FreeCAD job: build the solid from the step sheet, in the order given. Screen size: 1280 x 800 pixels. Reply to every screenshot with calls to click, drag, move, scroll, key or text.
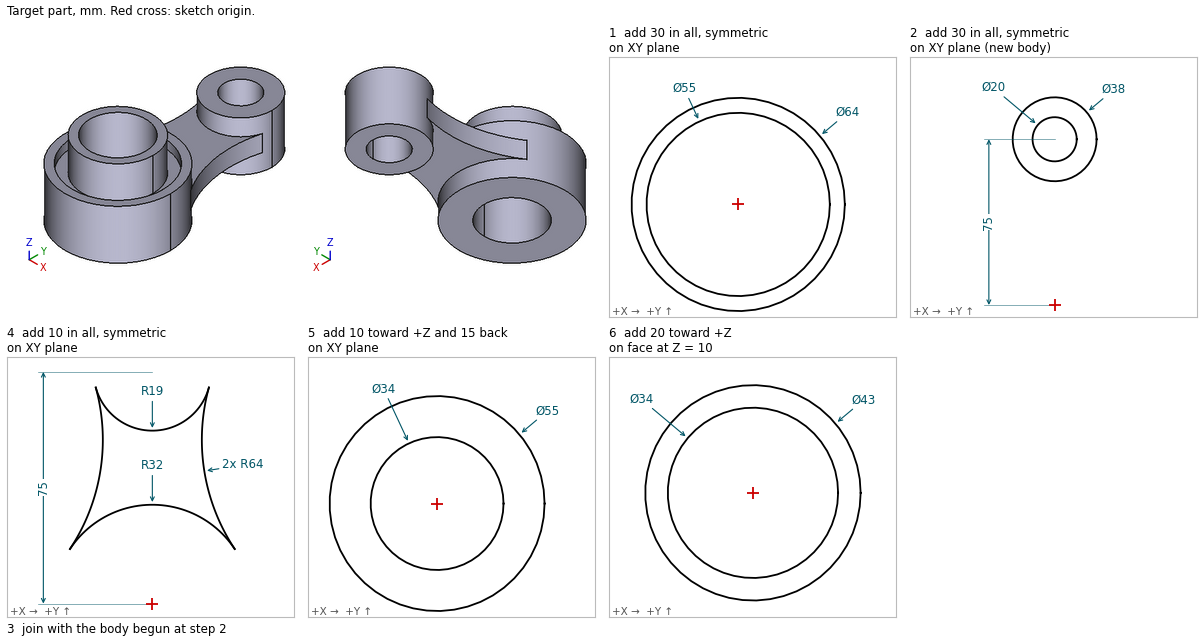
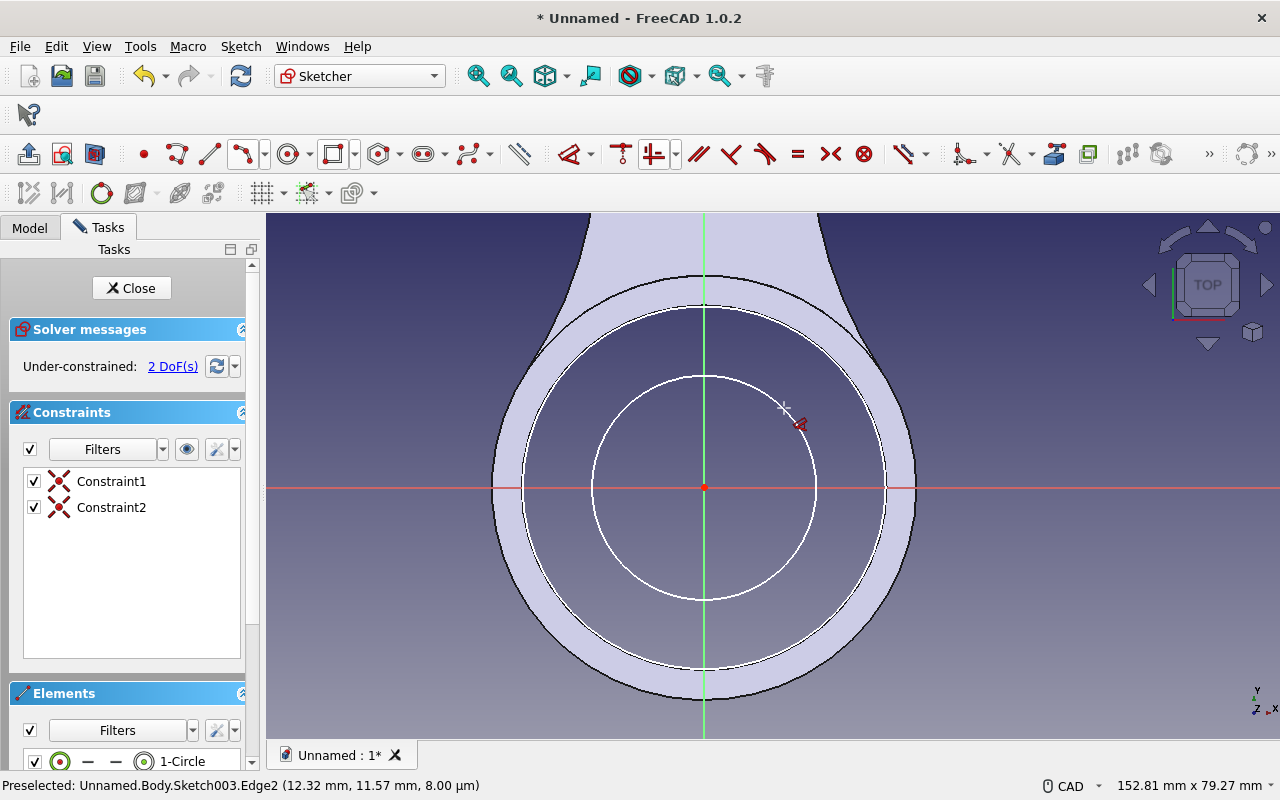
click(832, 359)
click(855, 336)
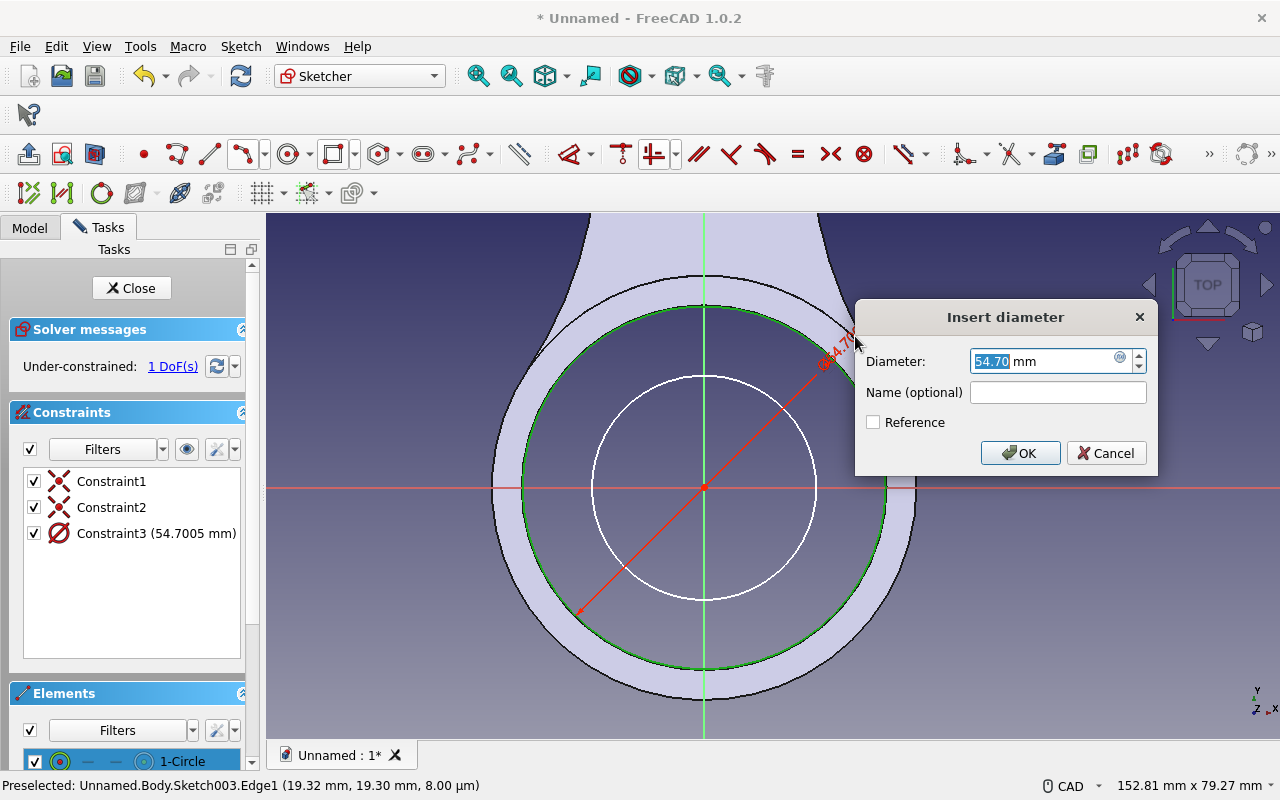
text(55)
key(Return)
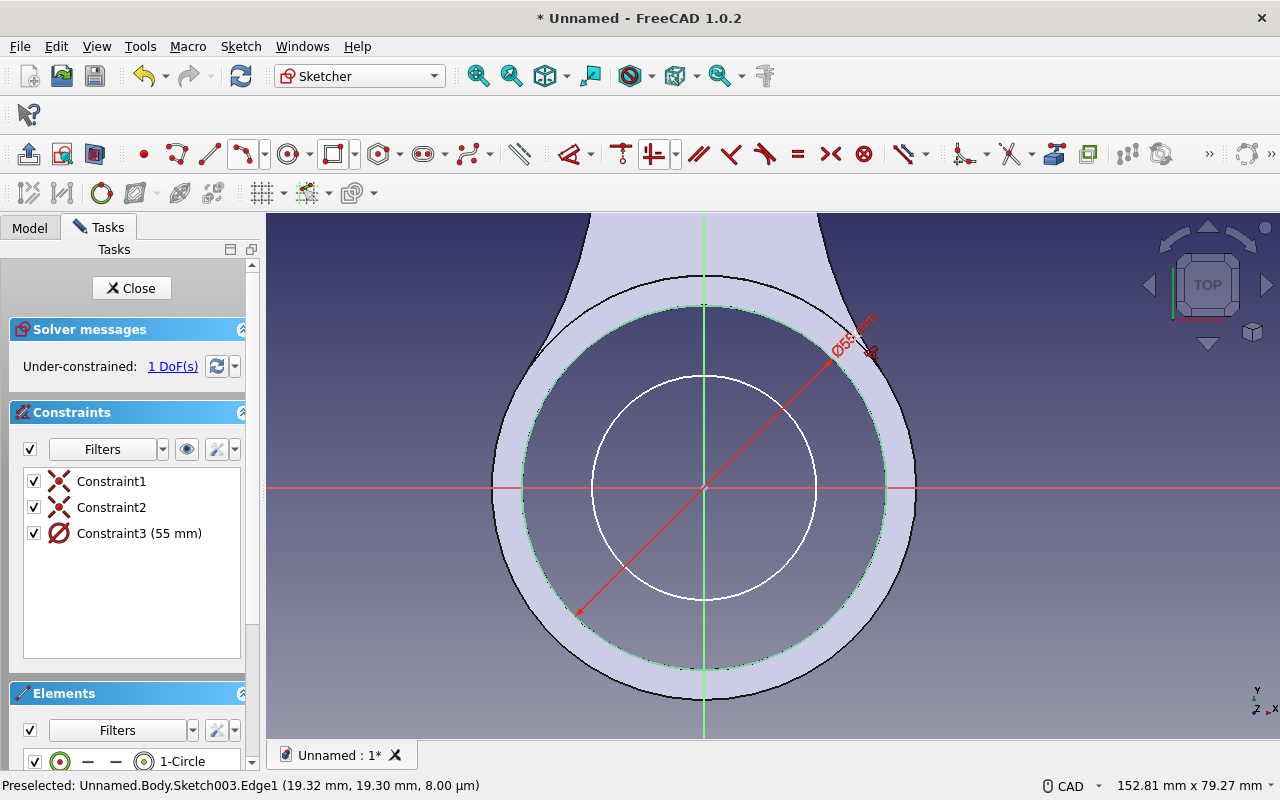
click(783, 408)
click(806, 385)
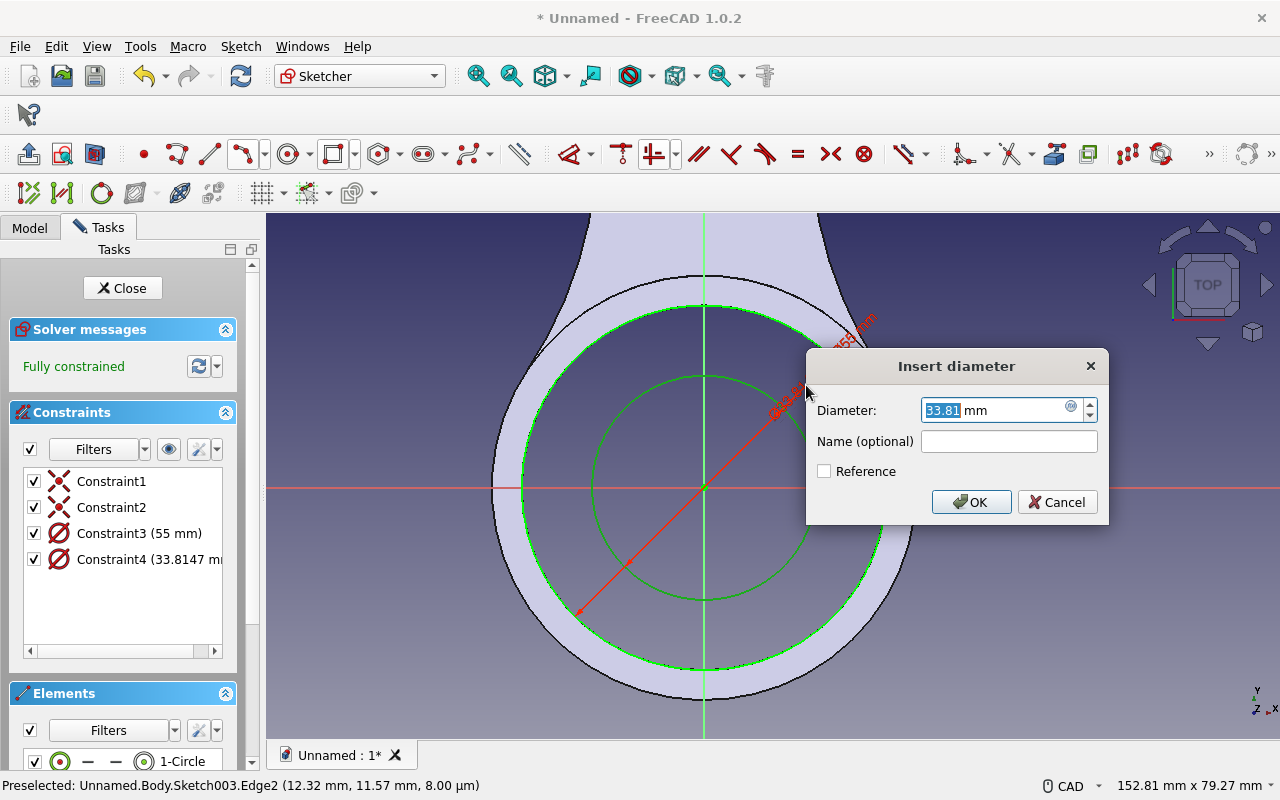
text(34)
key(Return)
key(Escape)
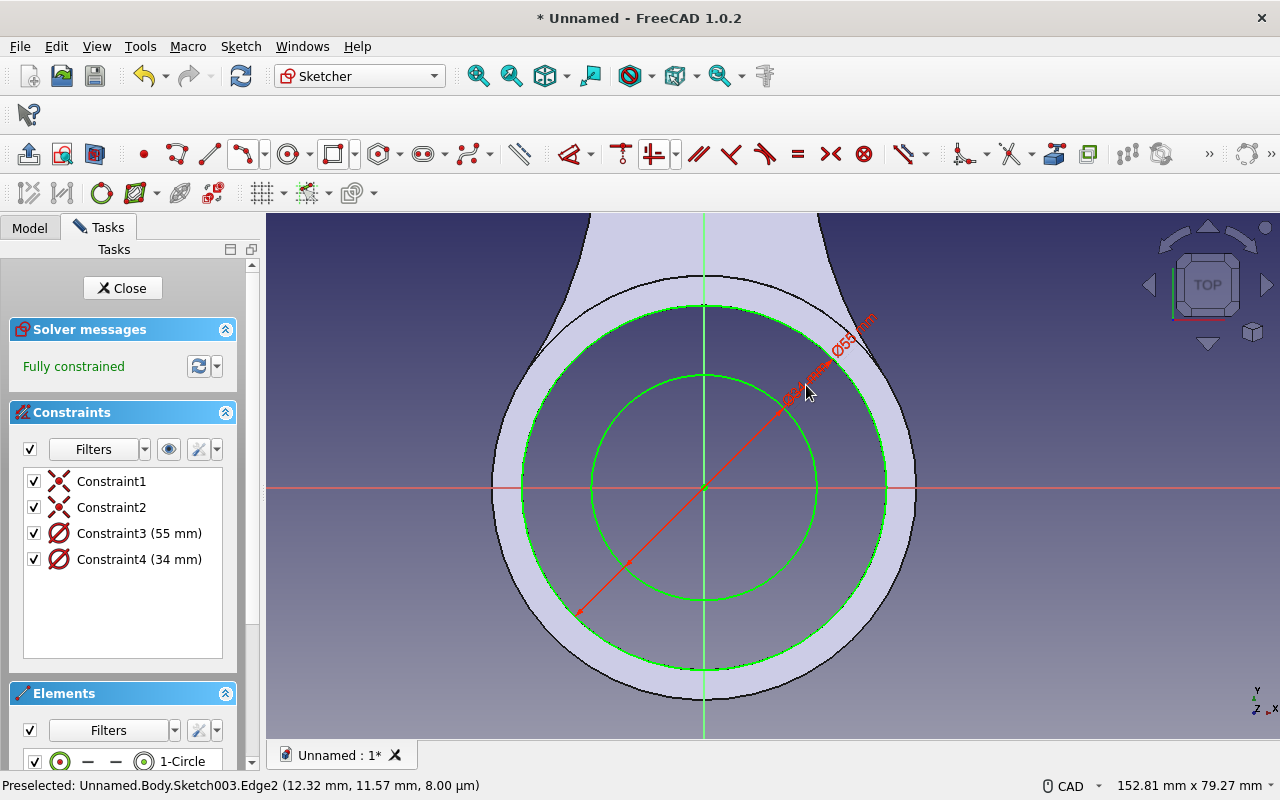
click(123, 288)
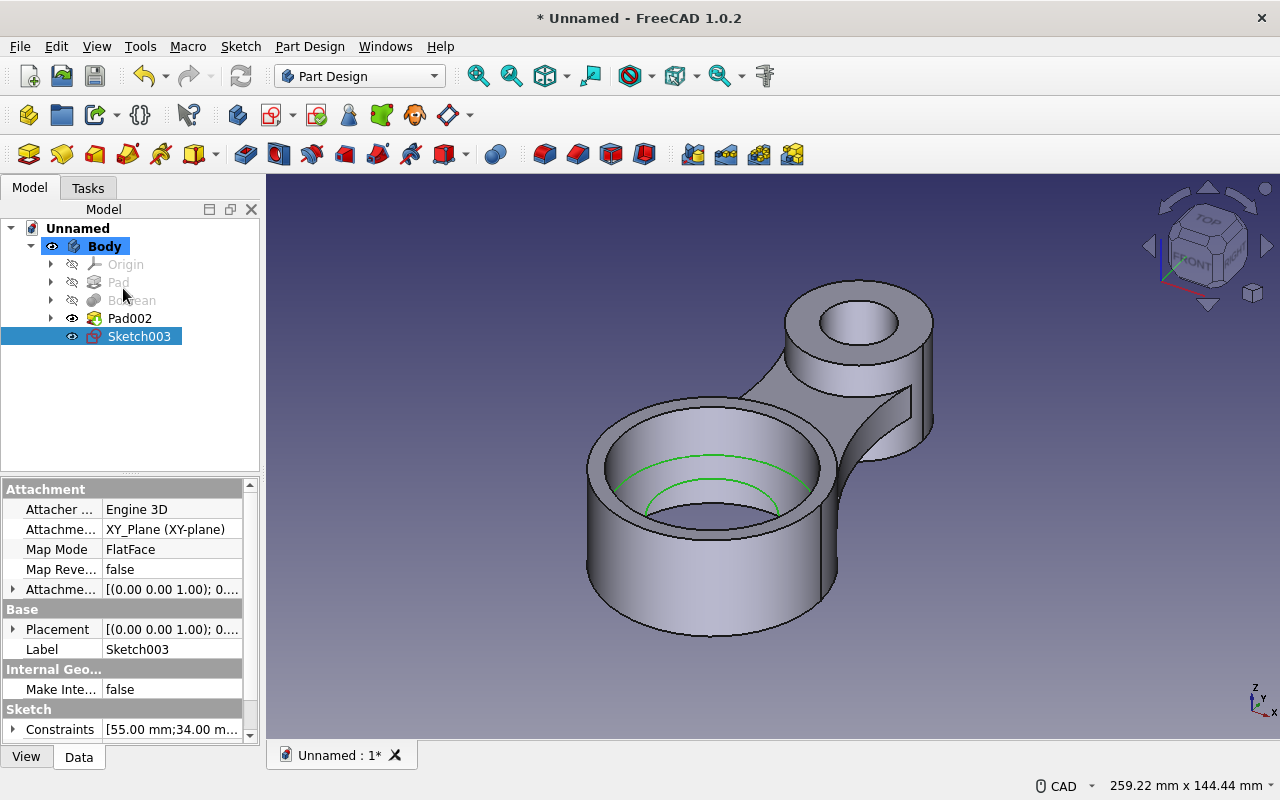
click(29, 154)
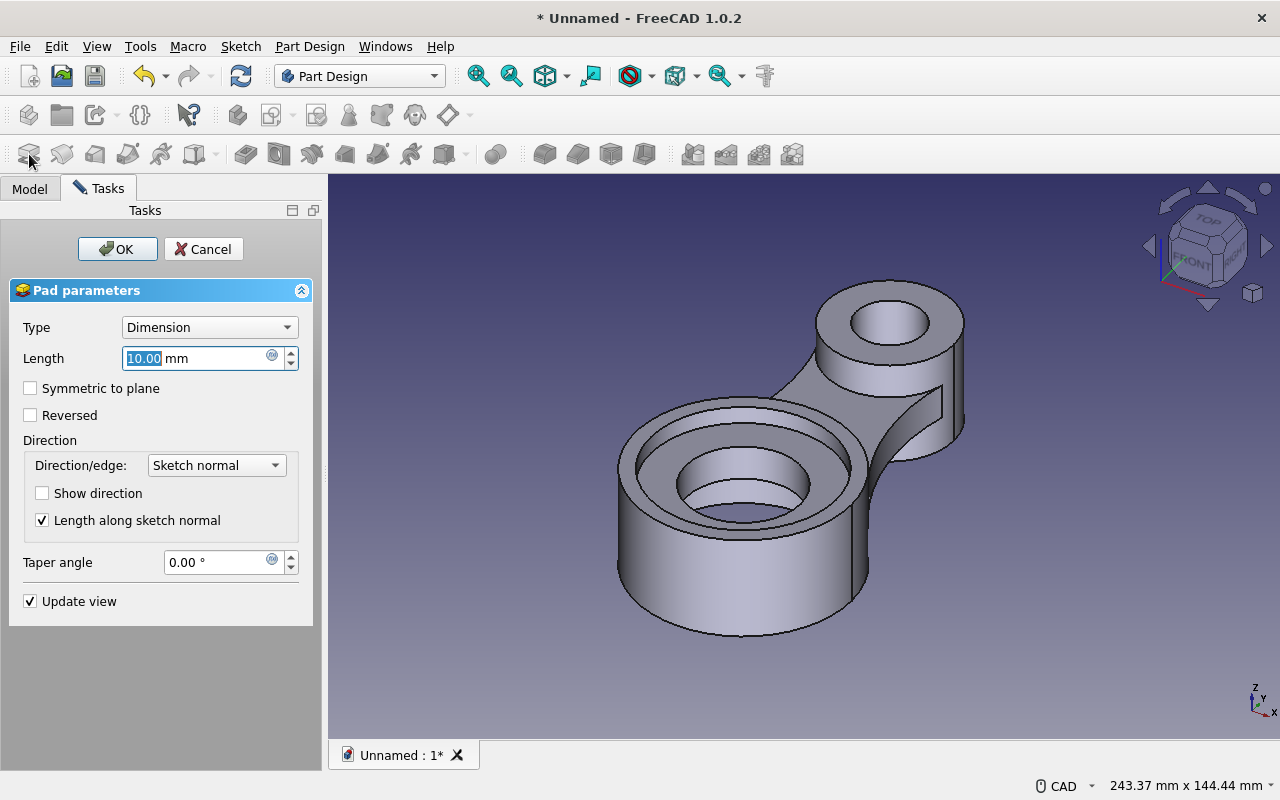
click(210, 328)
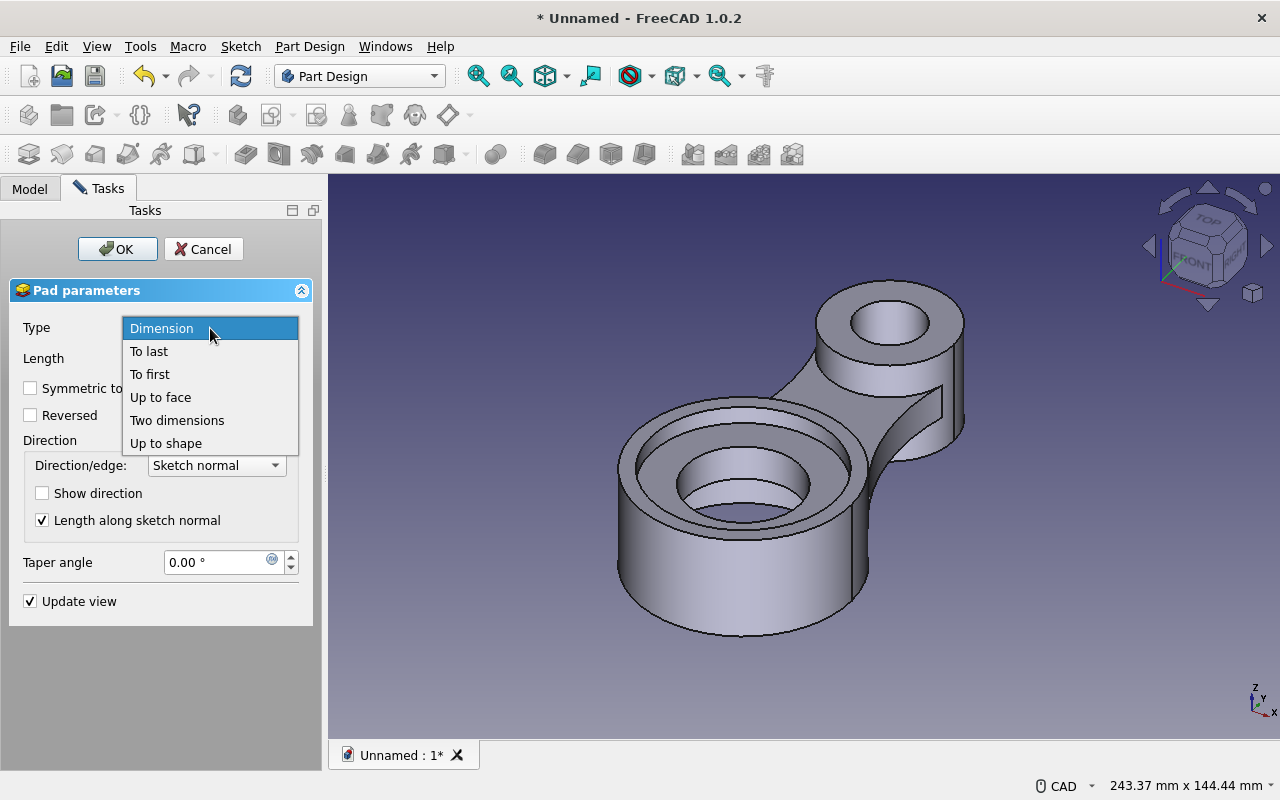
click(208, 420)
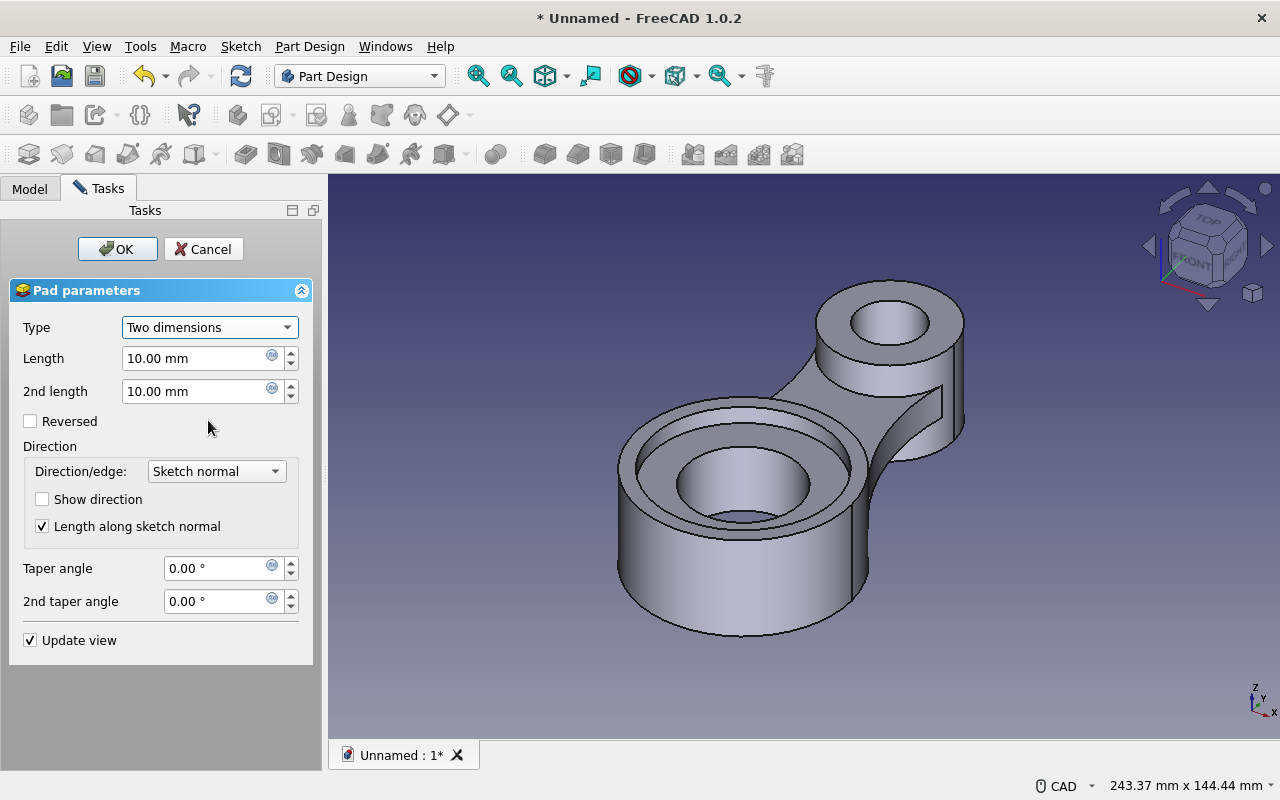
triple_click(204, 358)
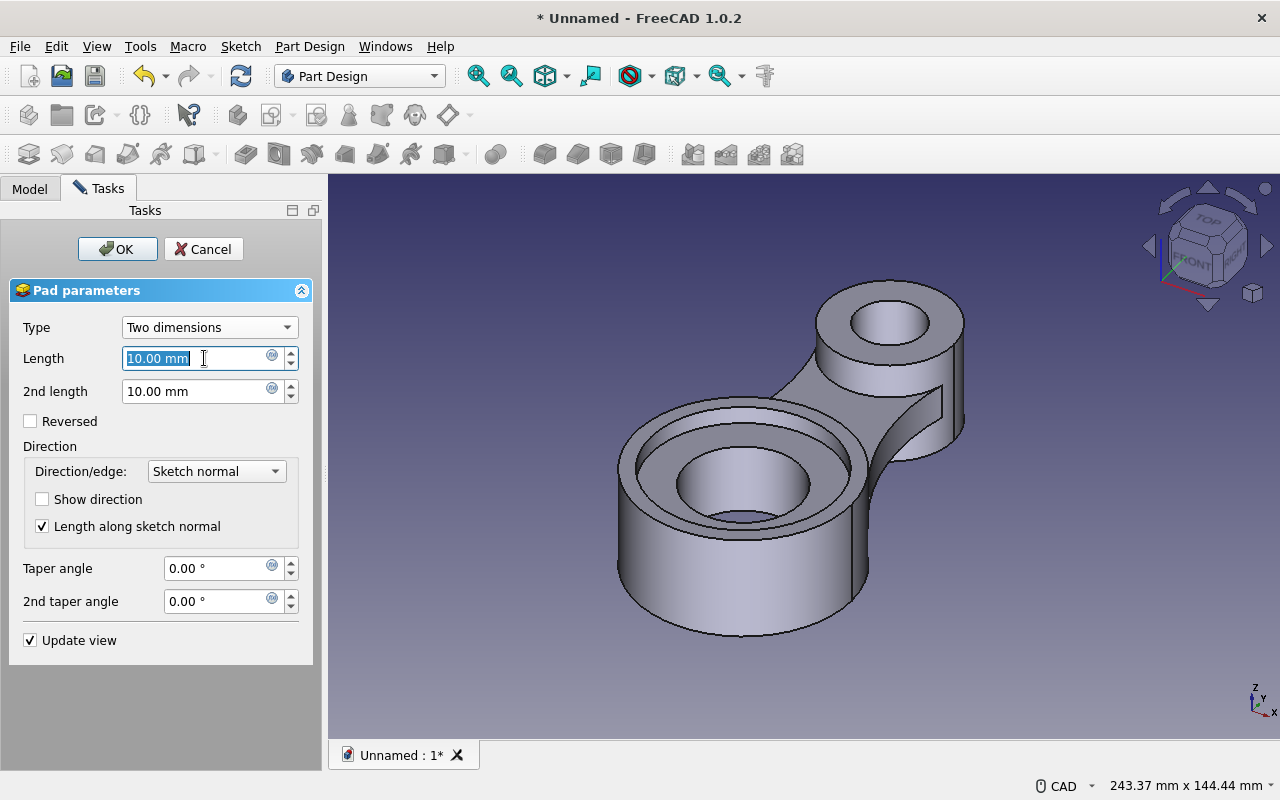
text(10)
key(Tab)